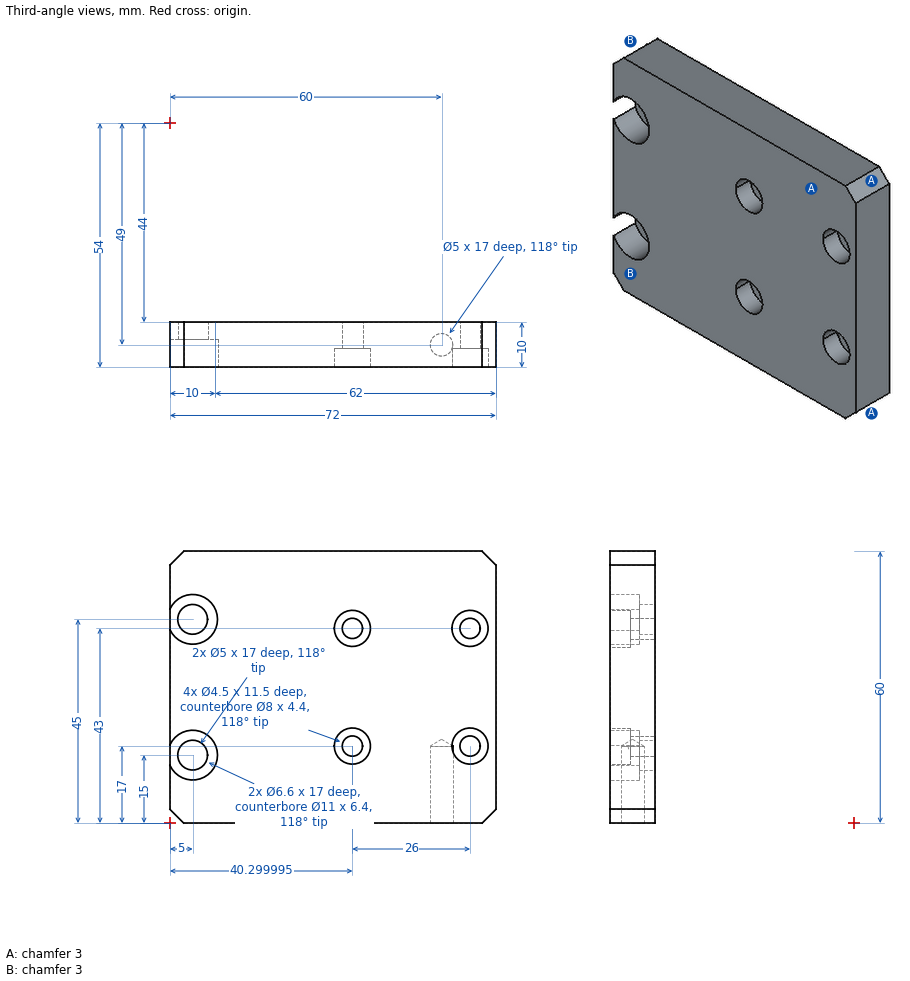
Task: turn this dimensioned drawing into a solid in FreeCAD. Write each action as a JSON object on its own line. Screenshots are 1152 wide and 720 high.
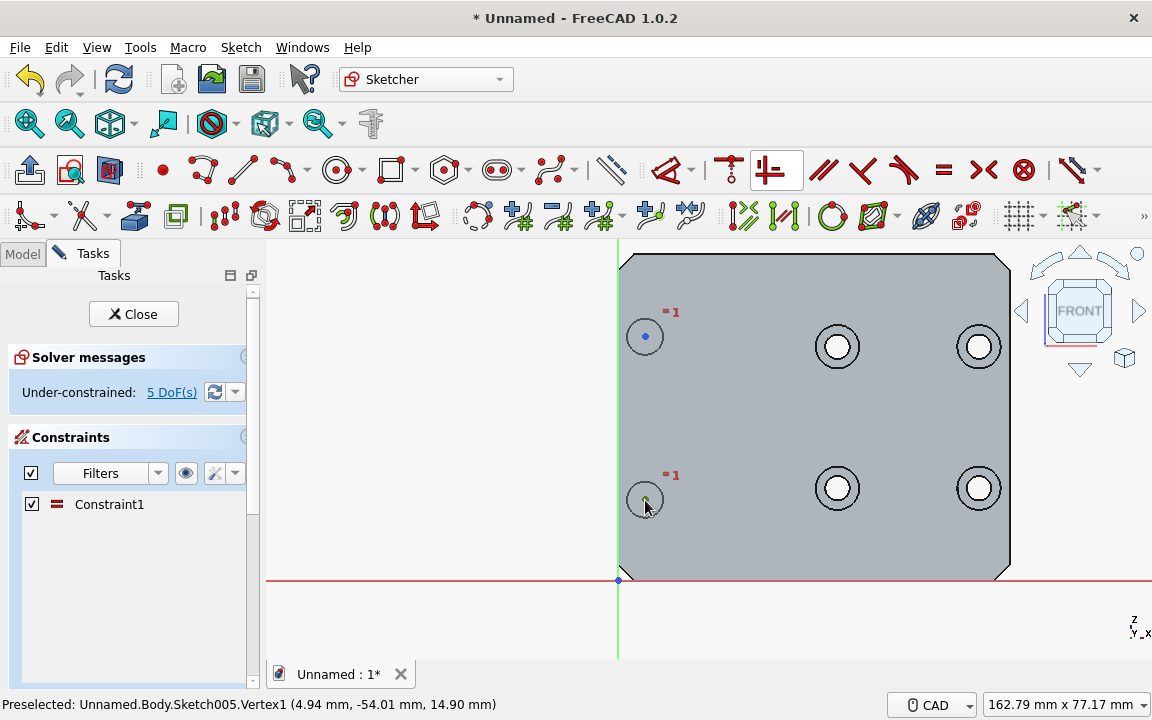
{"action": "left_click", "coordinate": [645, 337]}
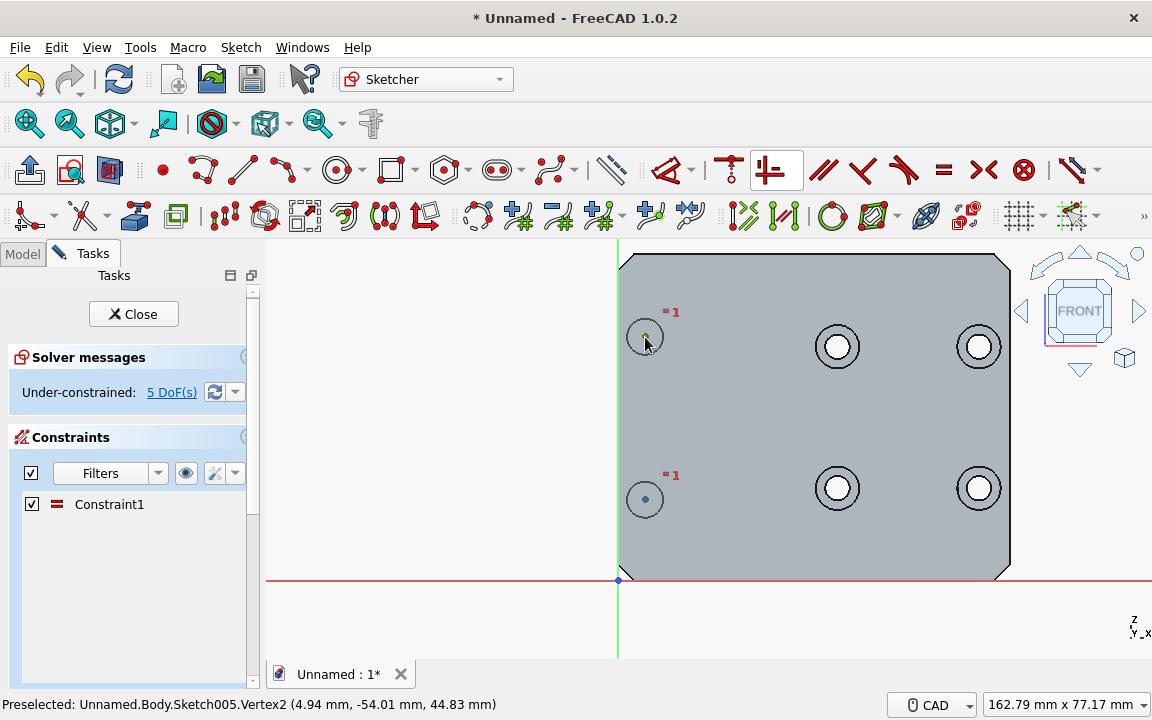
{"action": "left_click", "coordinate": [798, 170]}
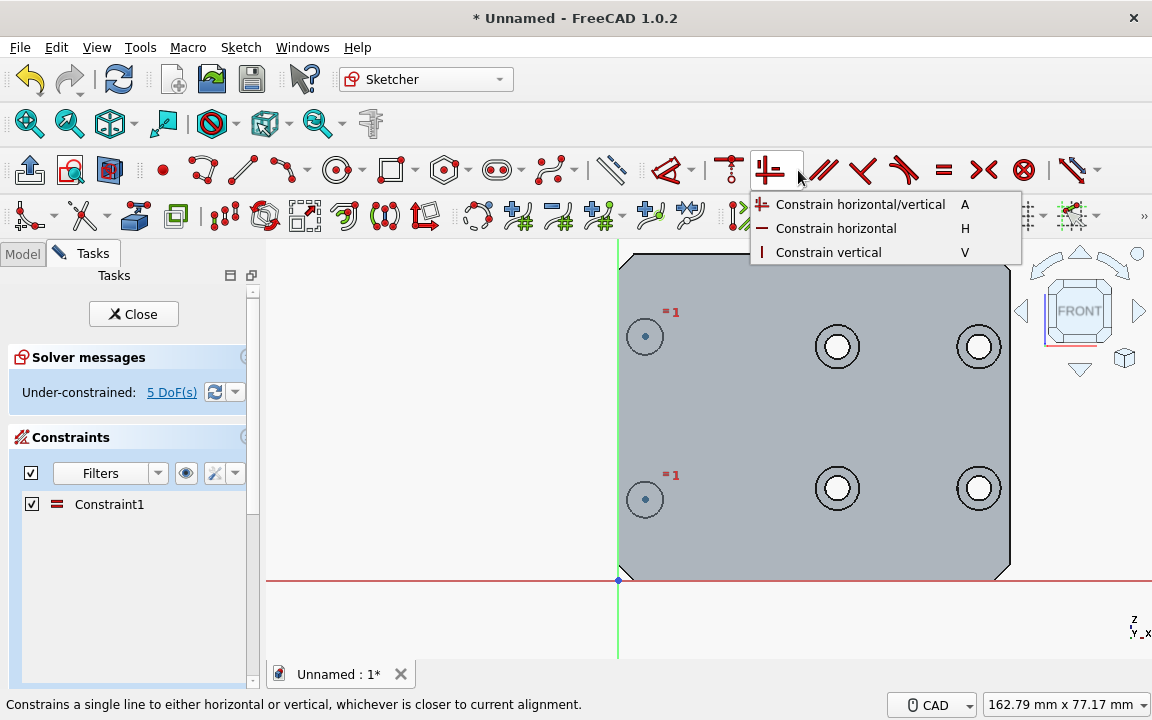
{"action": "left_click", "coordinate": [886, 252]}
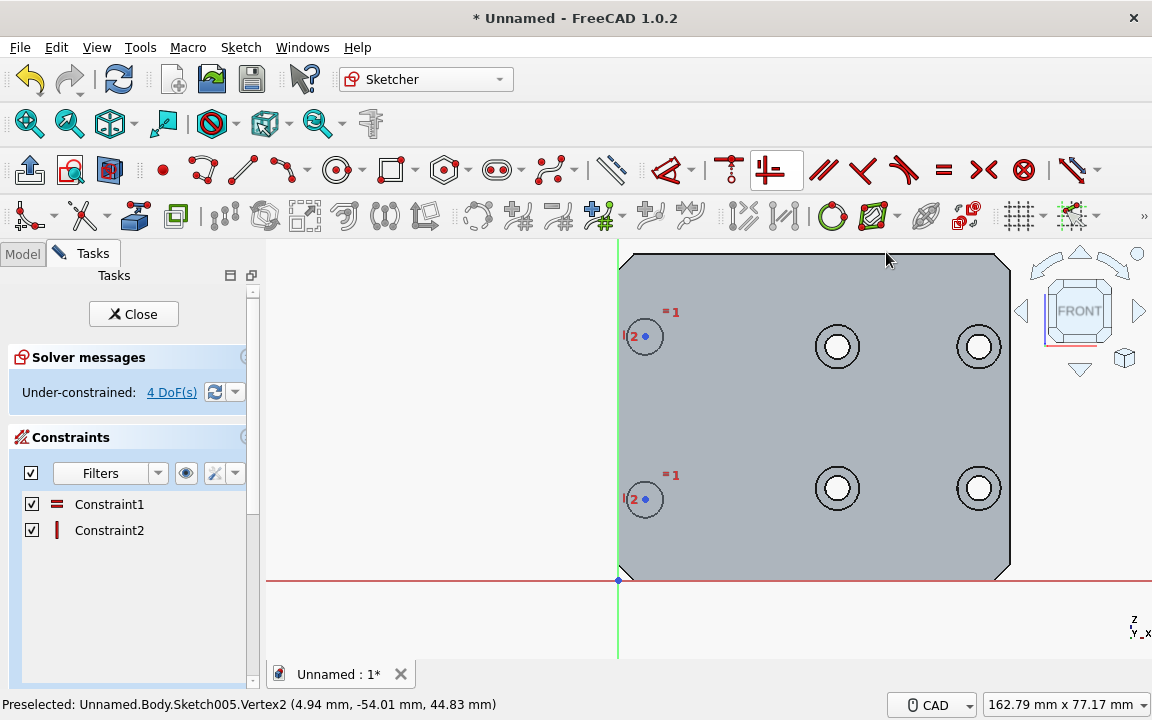
{"action": "left_click", "coordinate": [666, 170]}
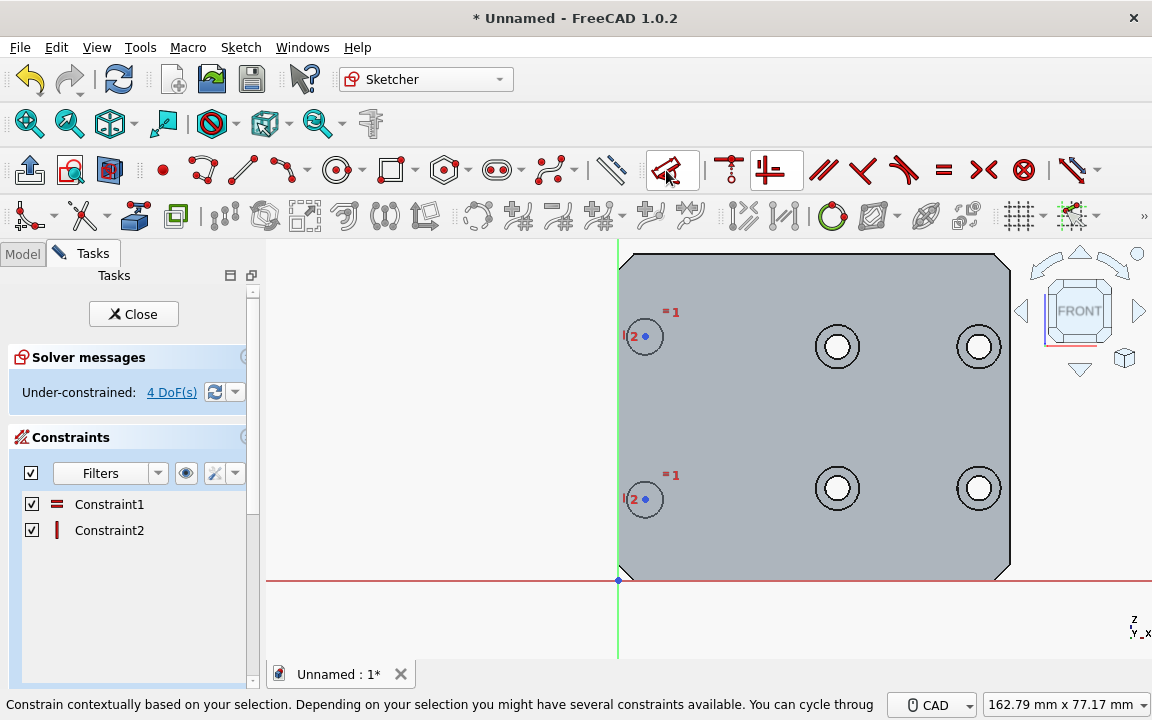
{"action": "left_click", "coordinate": [658, 487]}
{"action": "left_click", "coordinate": [681, 465]}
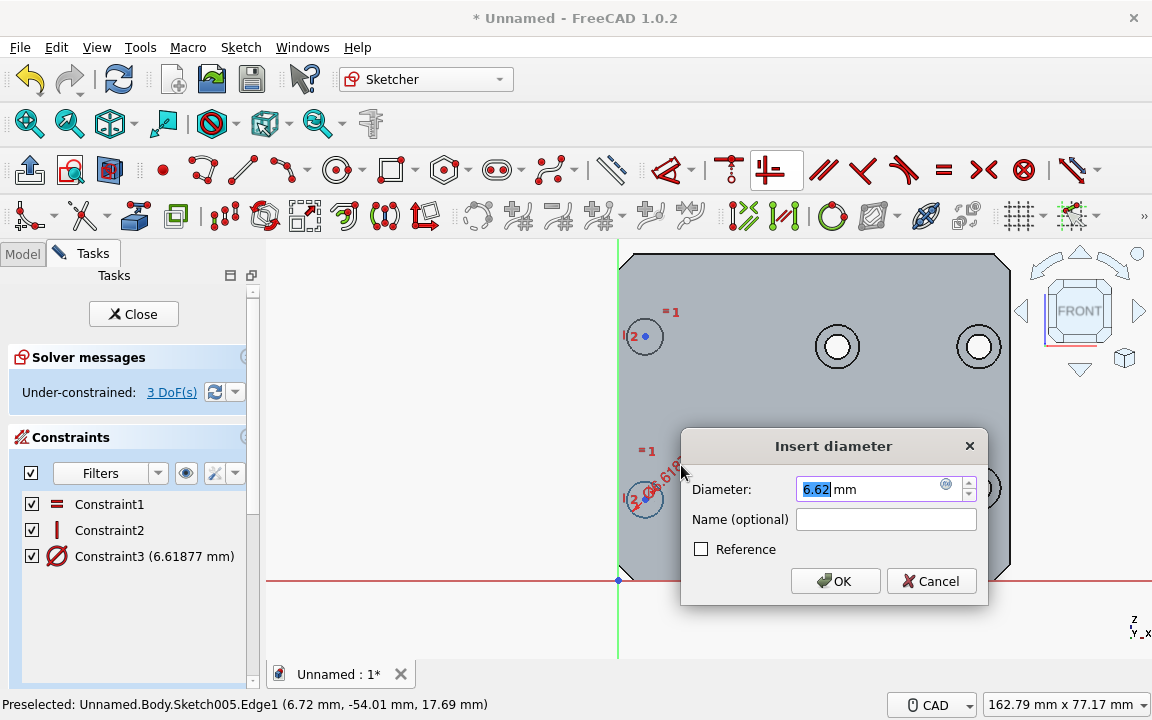
{"action": "type", "text": "6.6"}
{"action": "key", "text": "Return"}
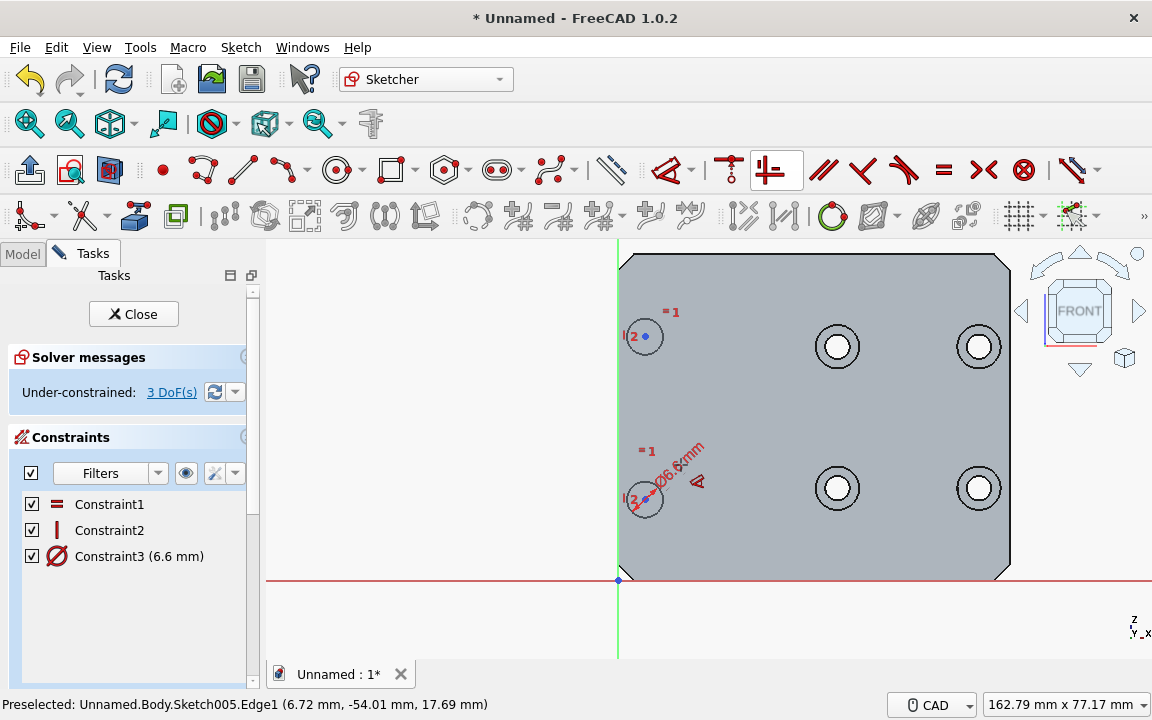
{"action": "scroll", "coordinate": [645, 500], "scroll_direction": "up", "scroll_amount": 2}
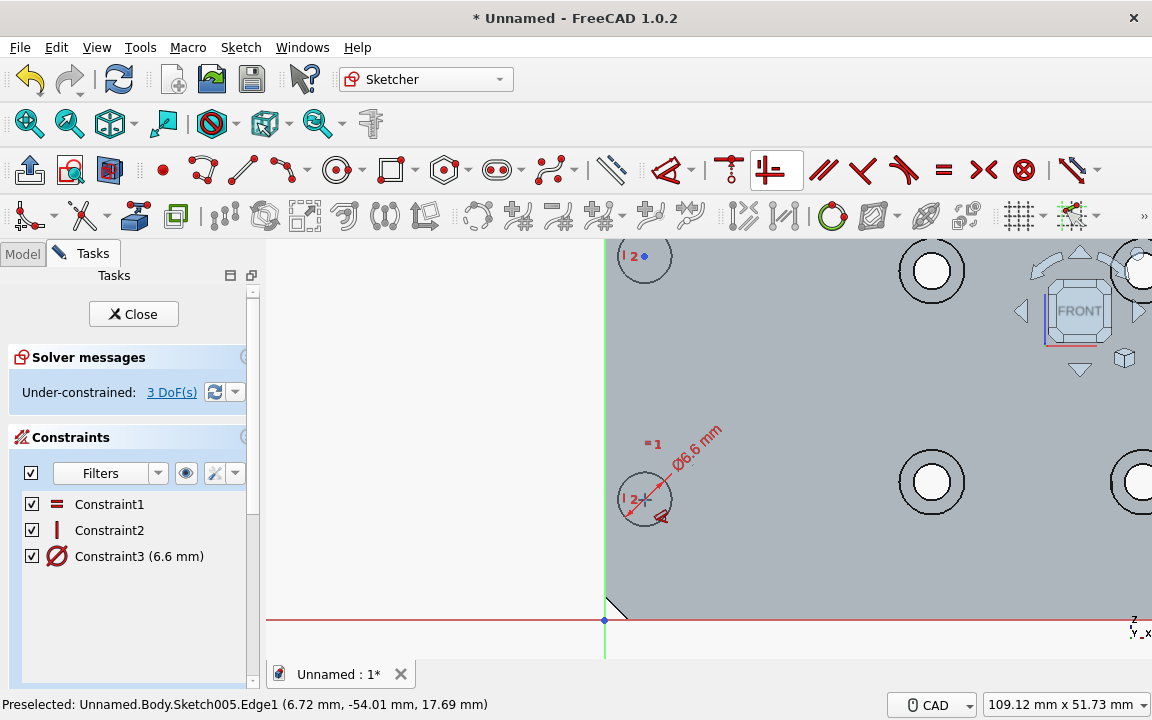
{"action": "left_click", "coordinate": [645, 499]}
{"action": "left_click", "coordinate": [625, 441]}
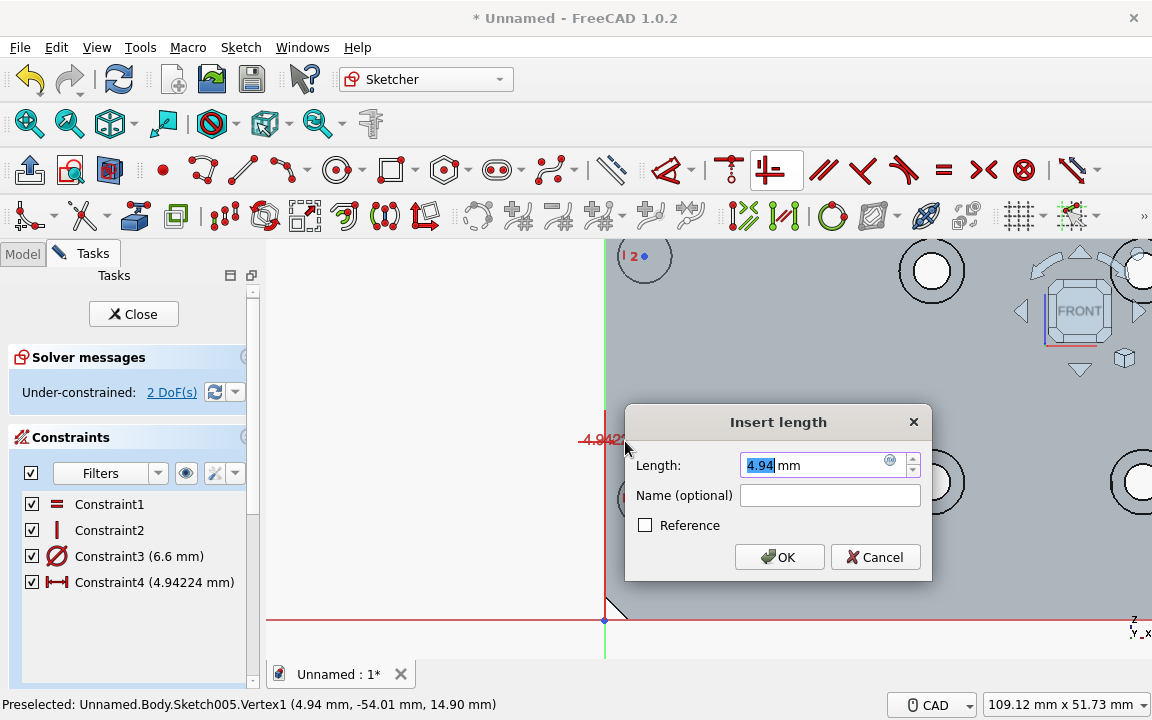
{"action": "type", "text": "5"}
{"action": "key", "text": "Return"}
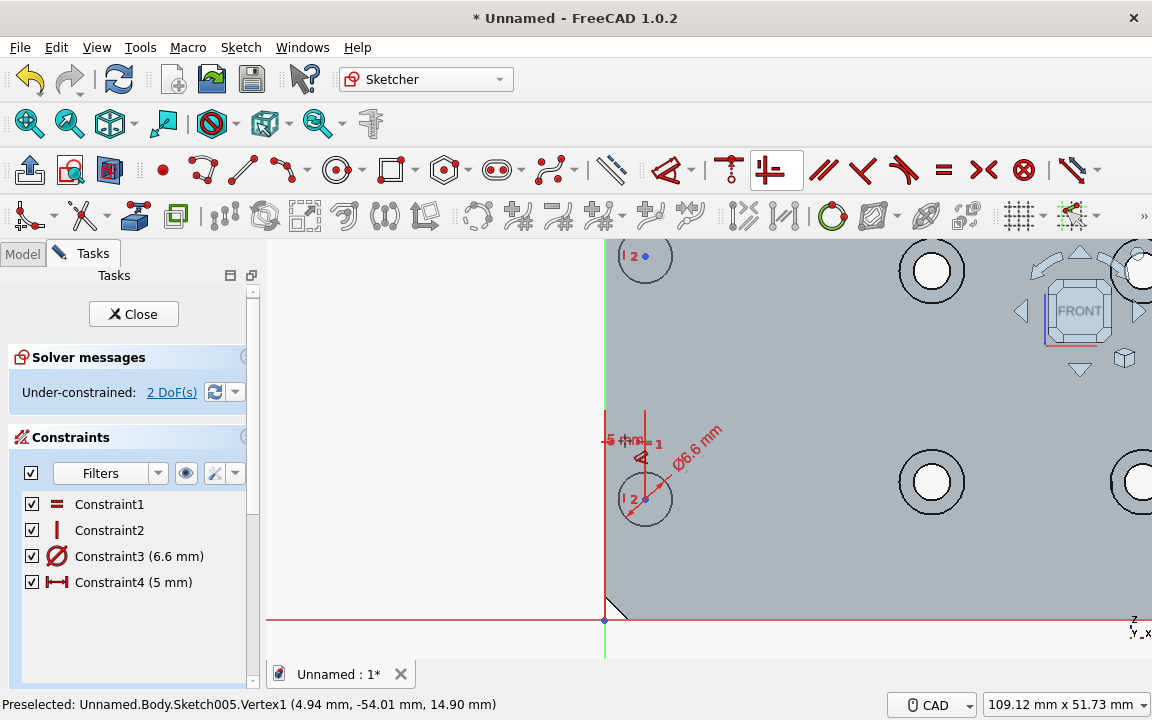
{"action": "left_click", "coordinate": [645, 499]}
{"action": "left_click", "coordinate": [571, 560]}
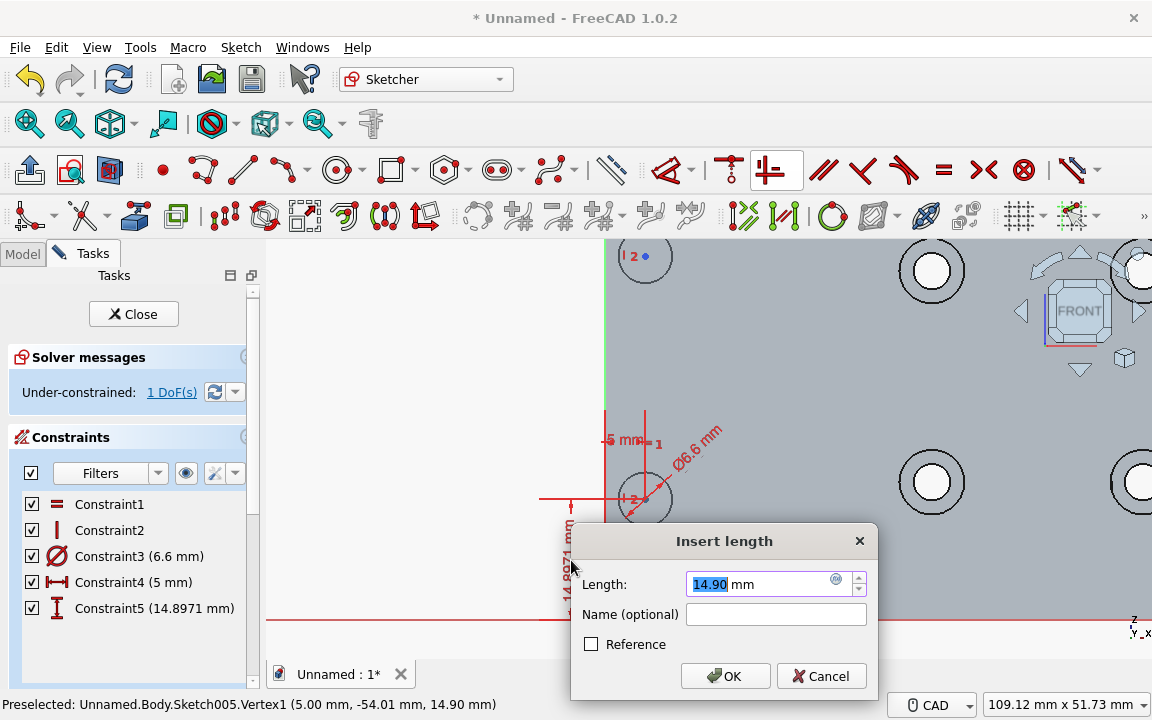
{"action": "type", "text": "15"}
{"action": "key", "text": "Return"}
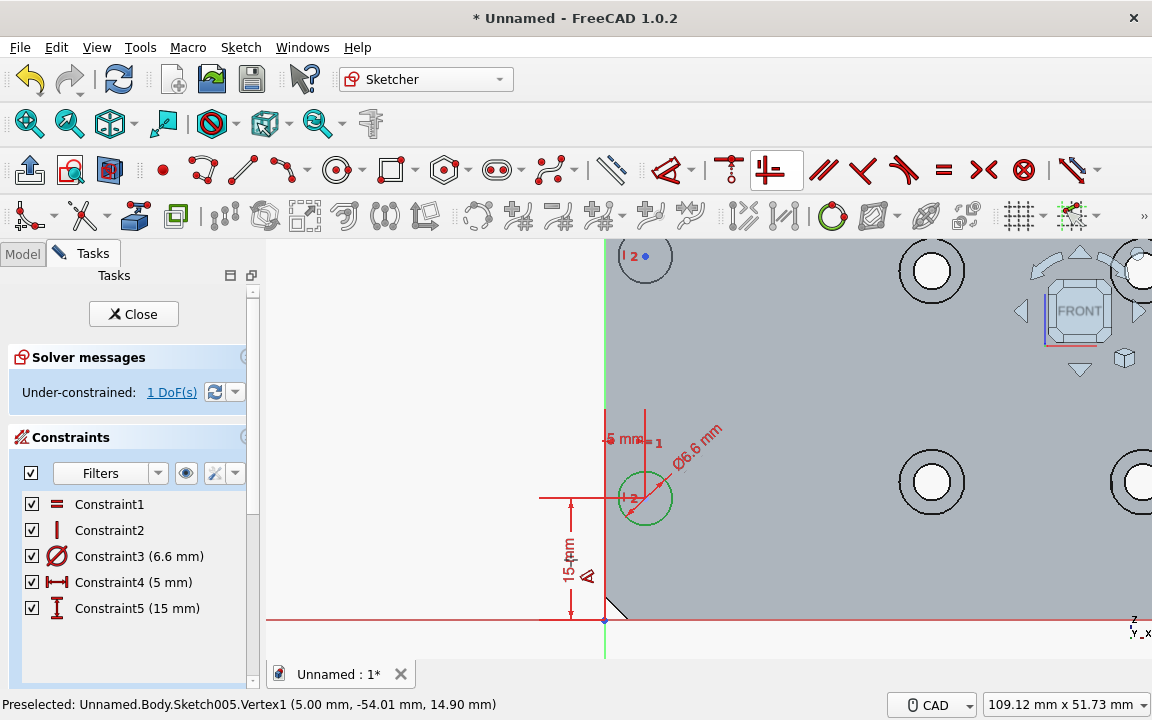
{"action": "scroll", "coordinate": [645, 500], "scroll_direction": "down", "scroll_amount": 2}